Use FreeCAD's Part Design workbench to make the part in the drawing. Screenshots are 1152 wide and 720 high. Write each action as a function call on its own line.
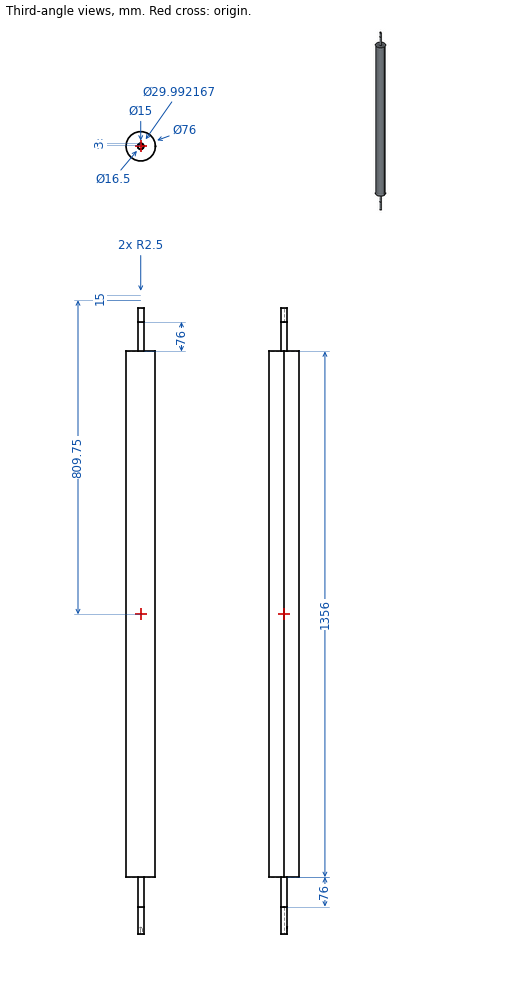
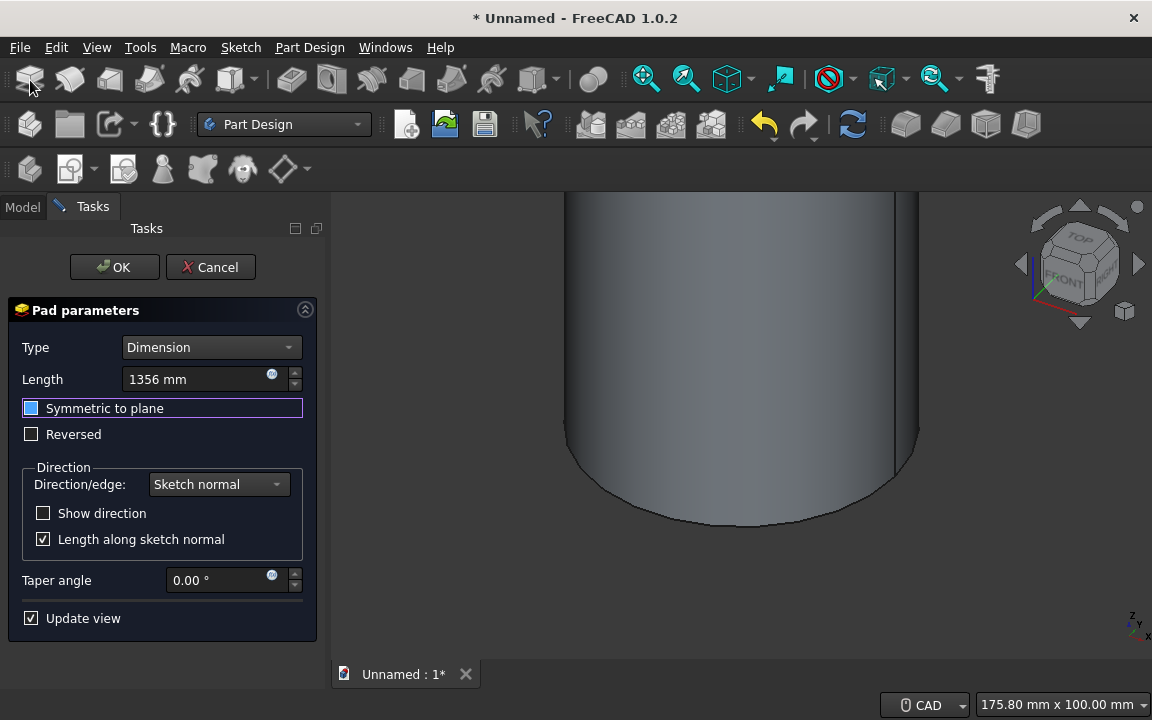
click(30, 408)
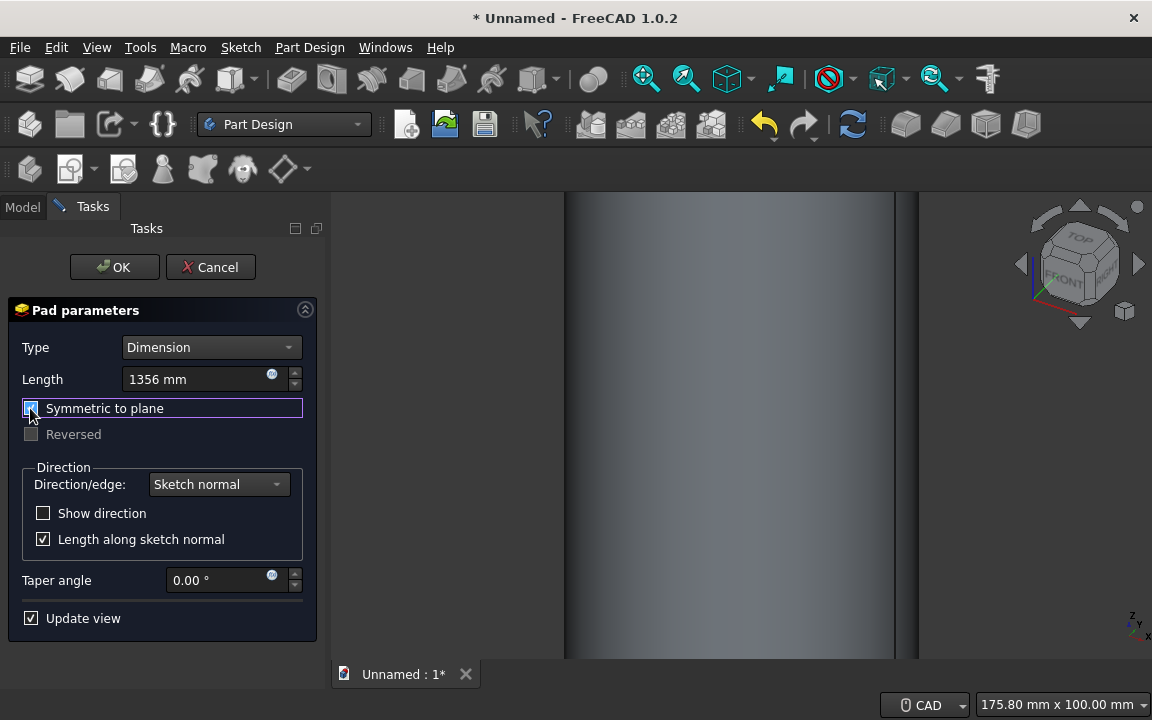
click(115, 267)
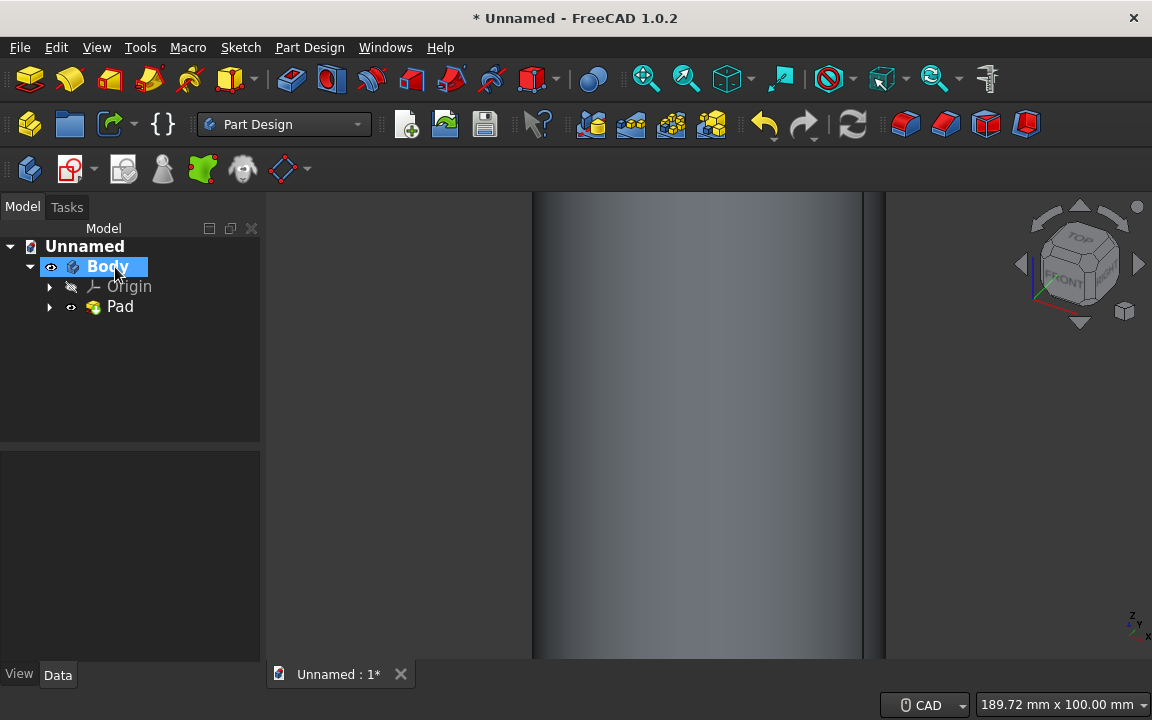
click(648, 80)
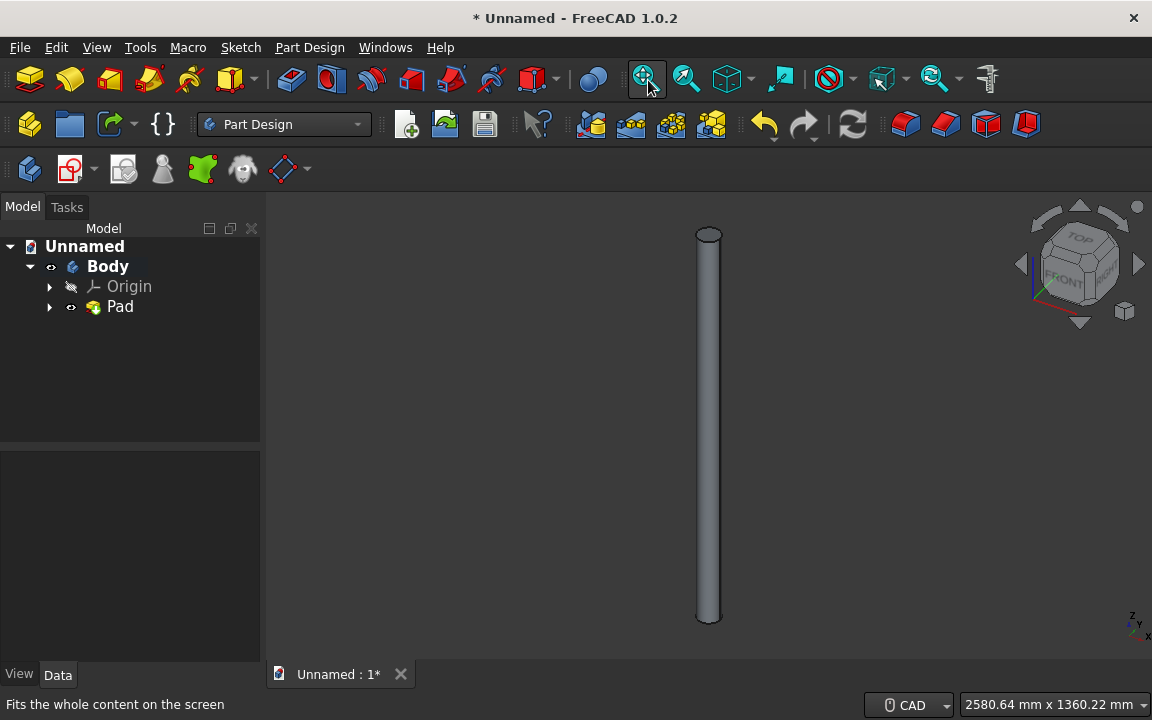
click(711, 232)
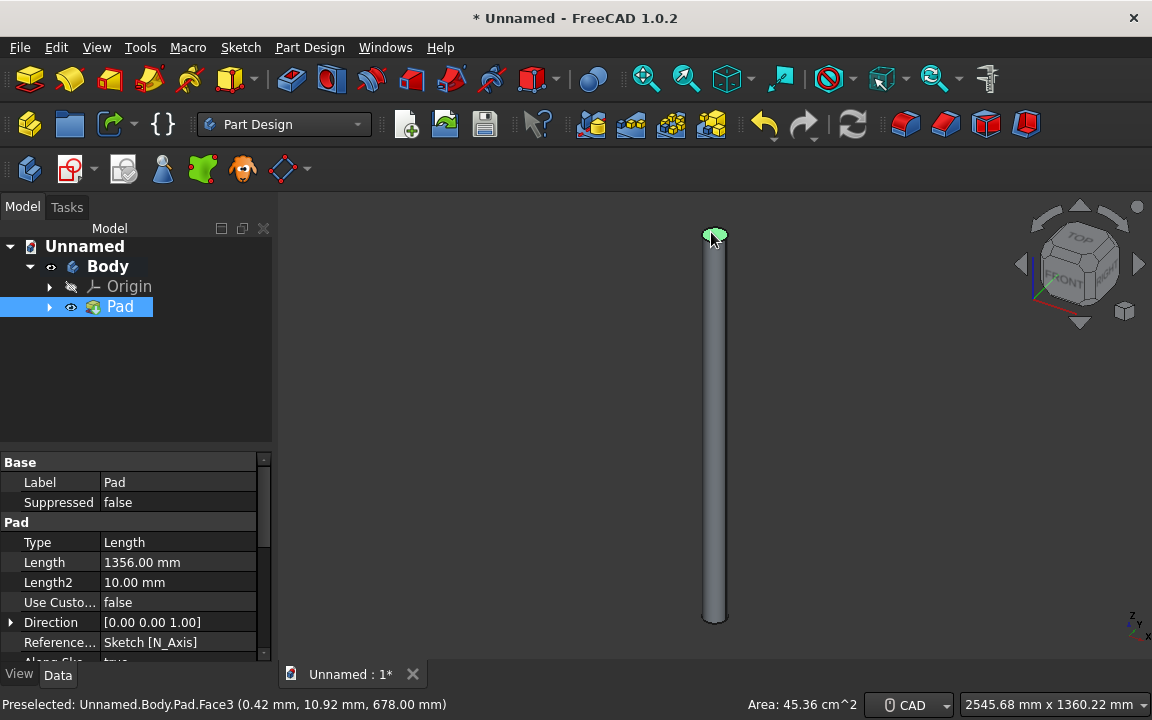
click(70, 170)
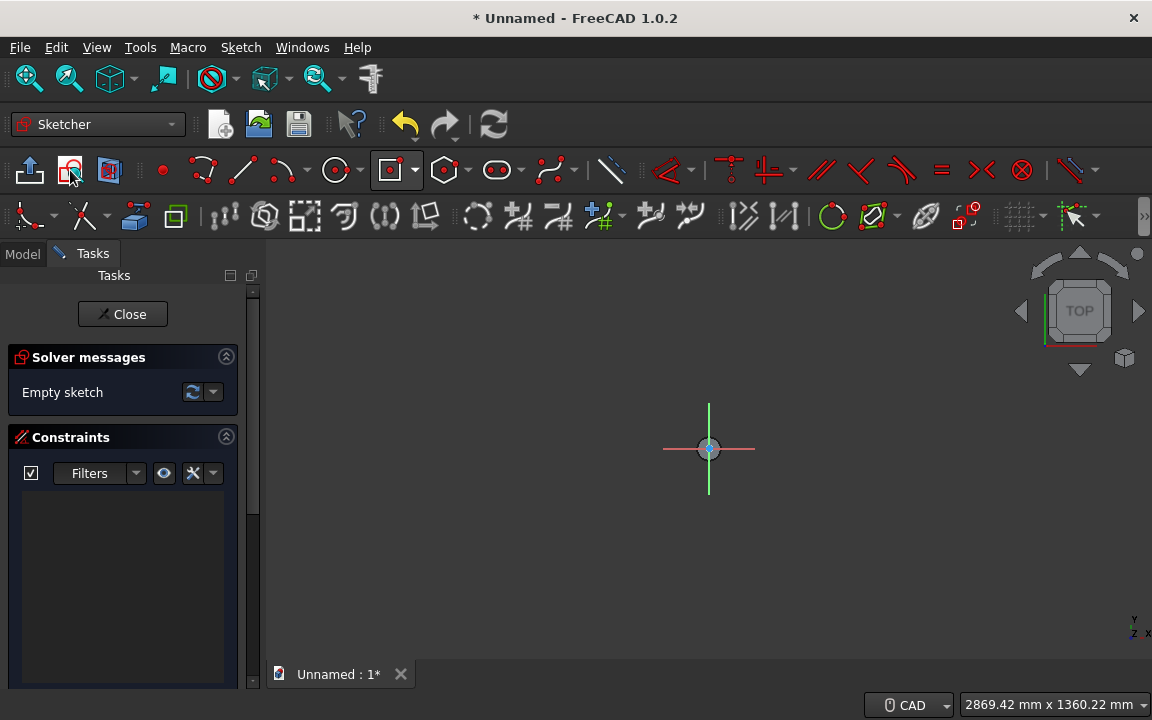
scroll(713, 449, up, 15)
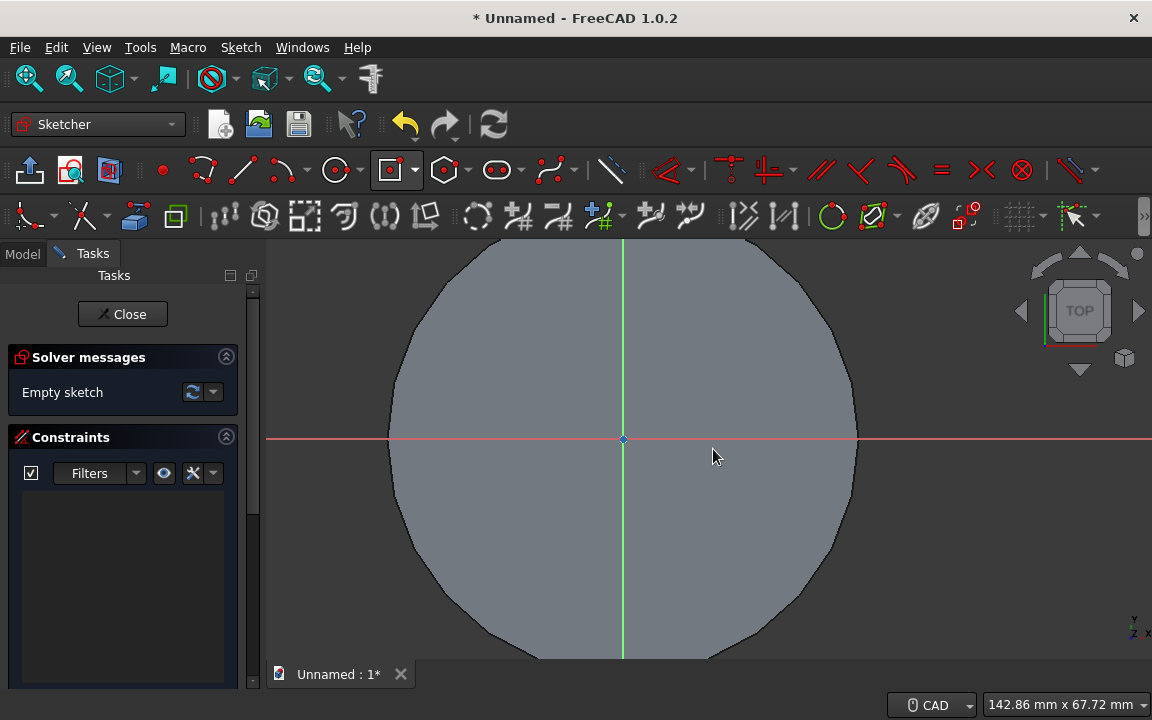
scroll(613, 434, up, 5)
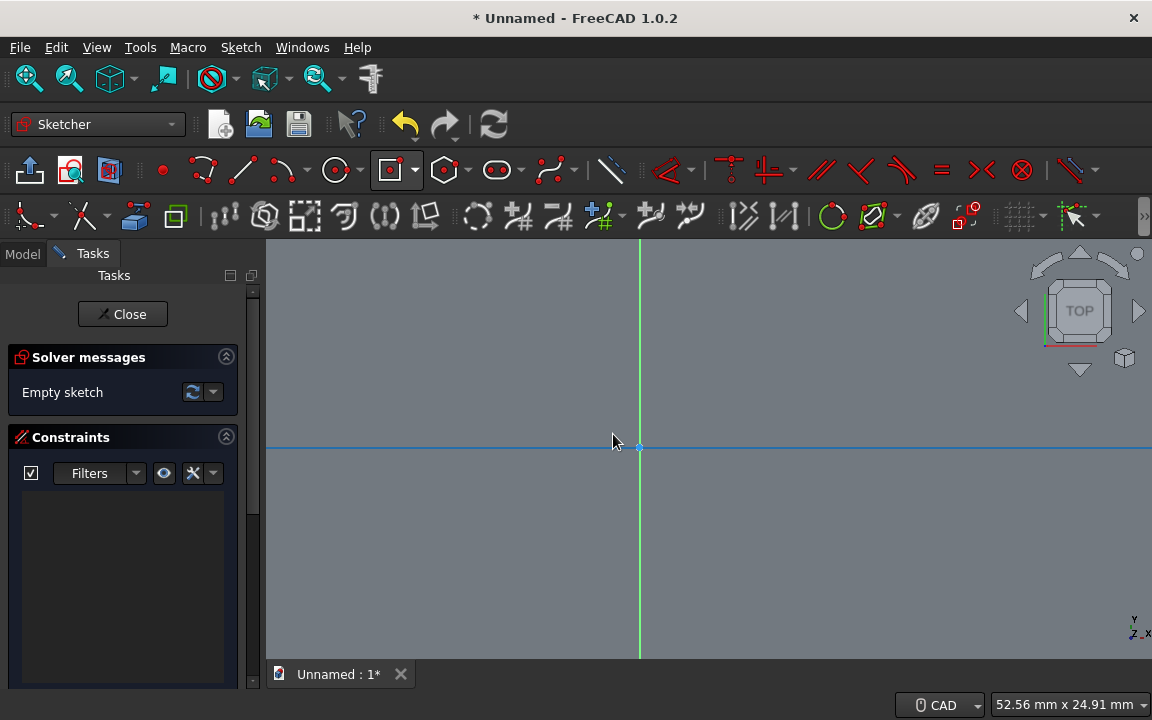
click(336, 170)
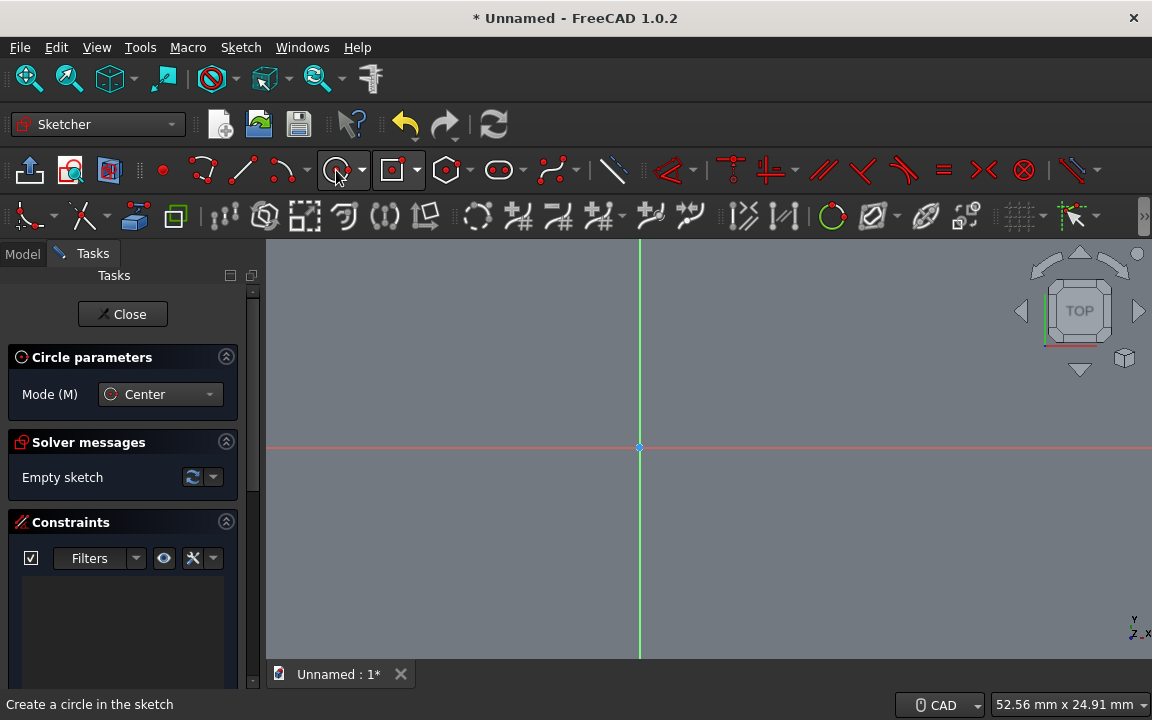
click(640, 448)
click(729, 359)
key(Escape)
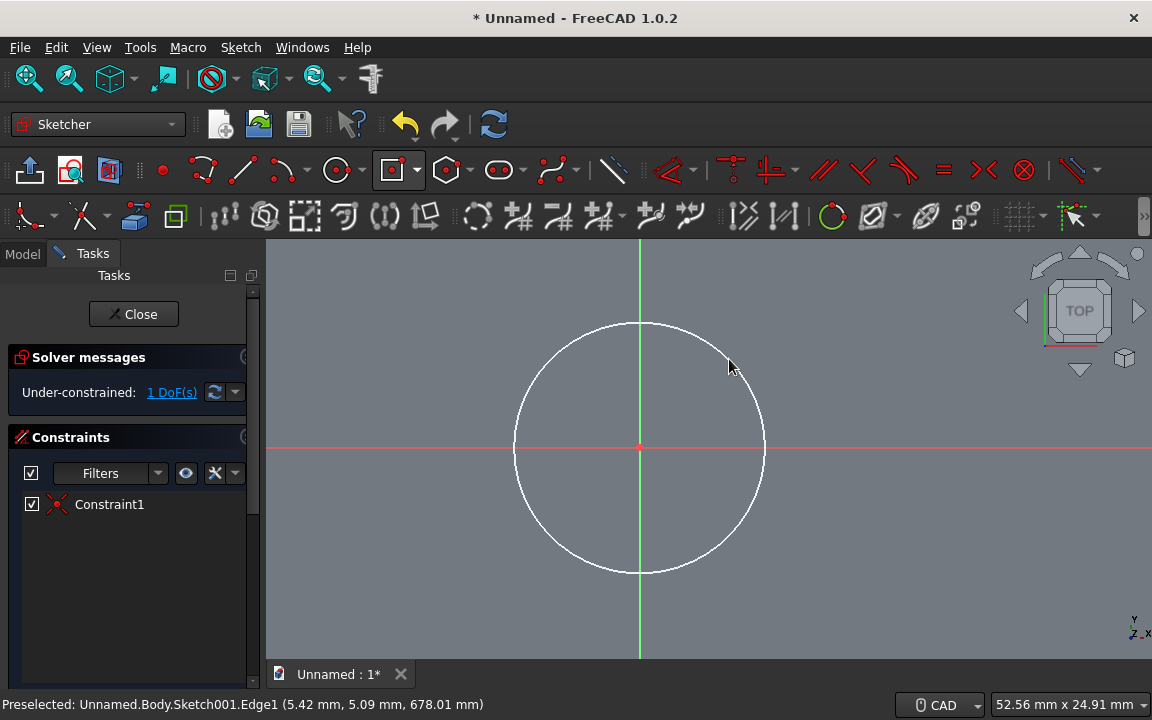
click(728, 359)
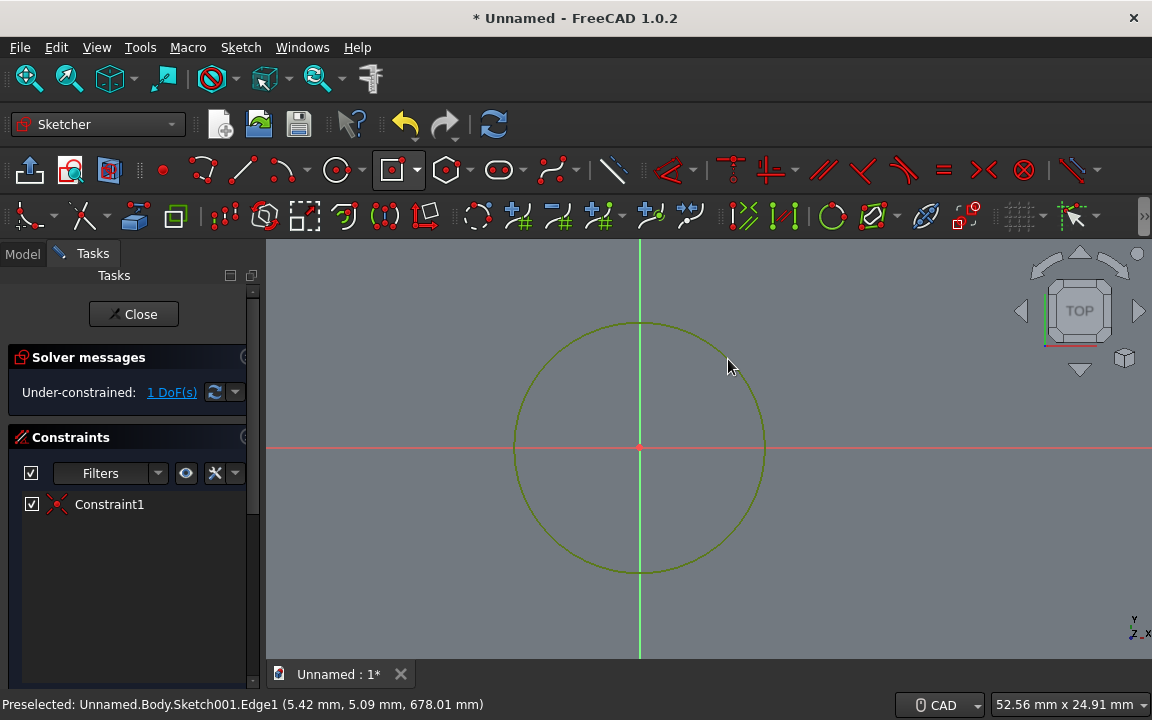
click(696, 170)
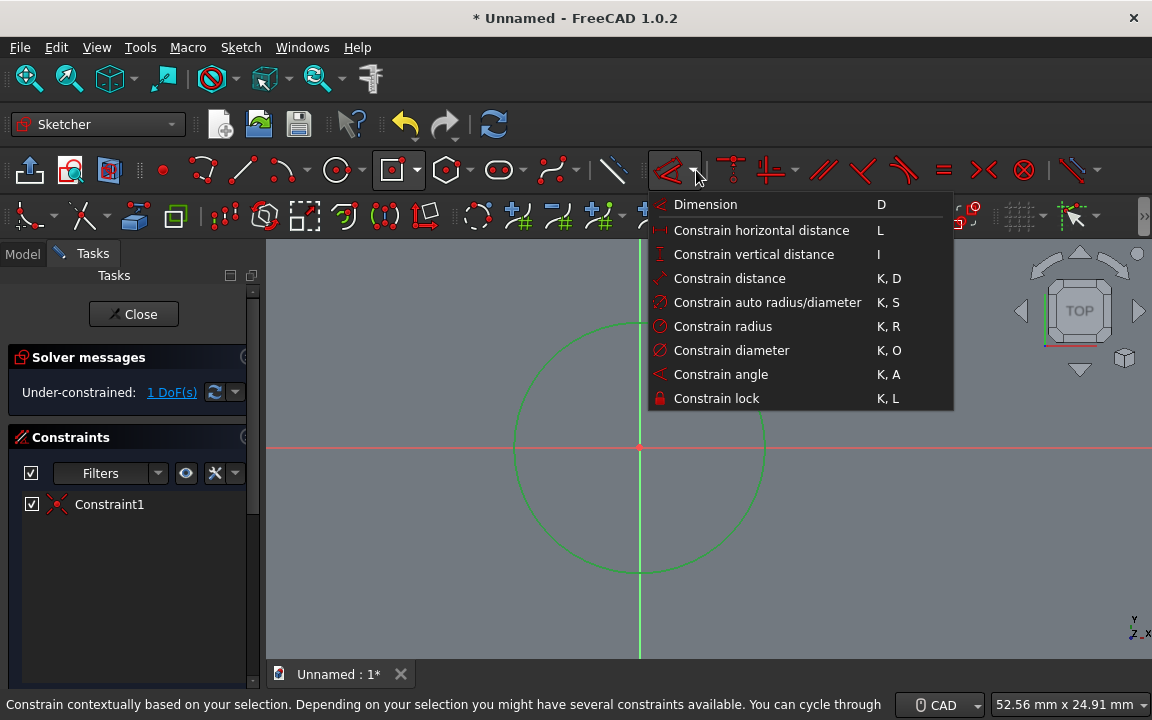
click(801, 350)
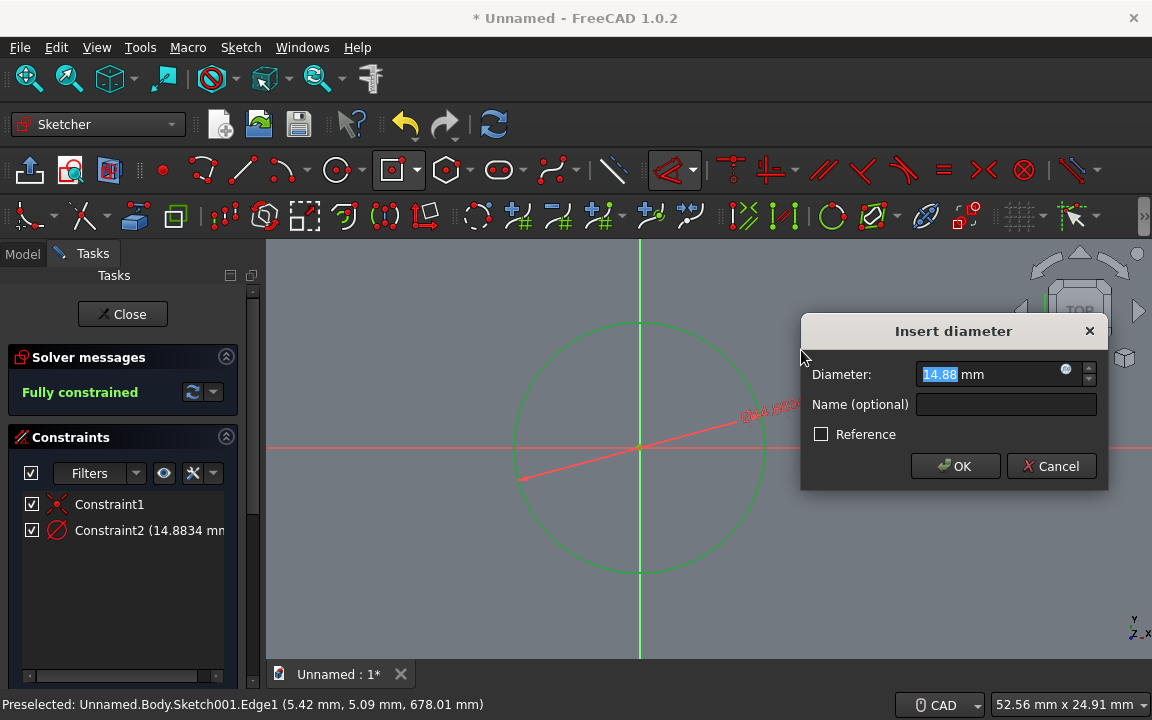
text(15)
key(Return)